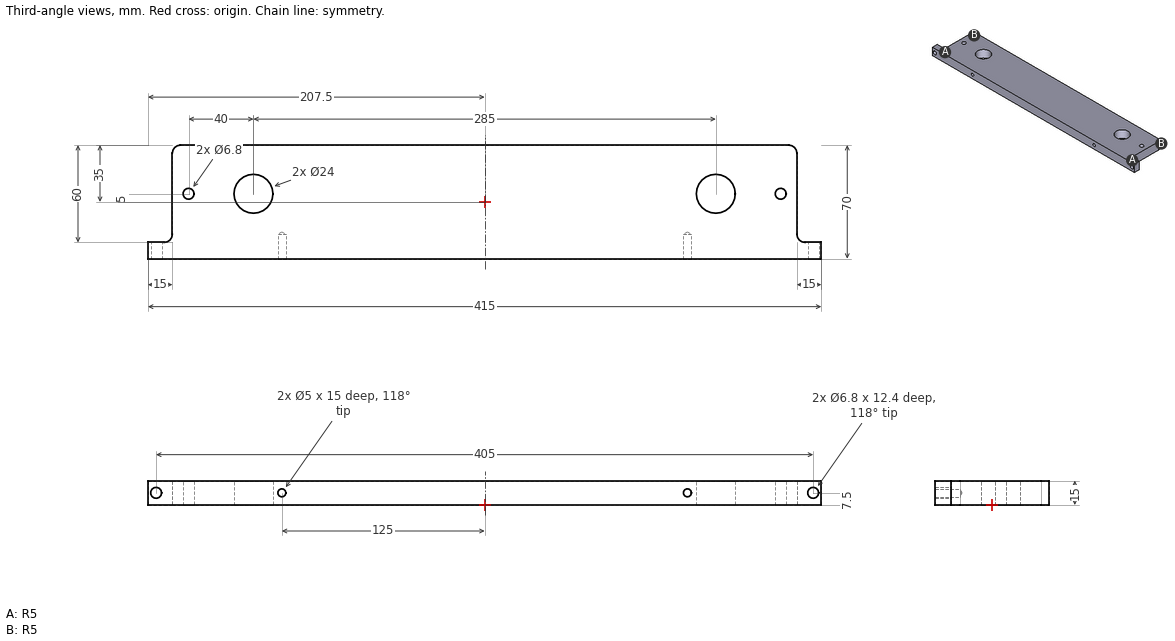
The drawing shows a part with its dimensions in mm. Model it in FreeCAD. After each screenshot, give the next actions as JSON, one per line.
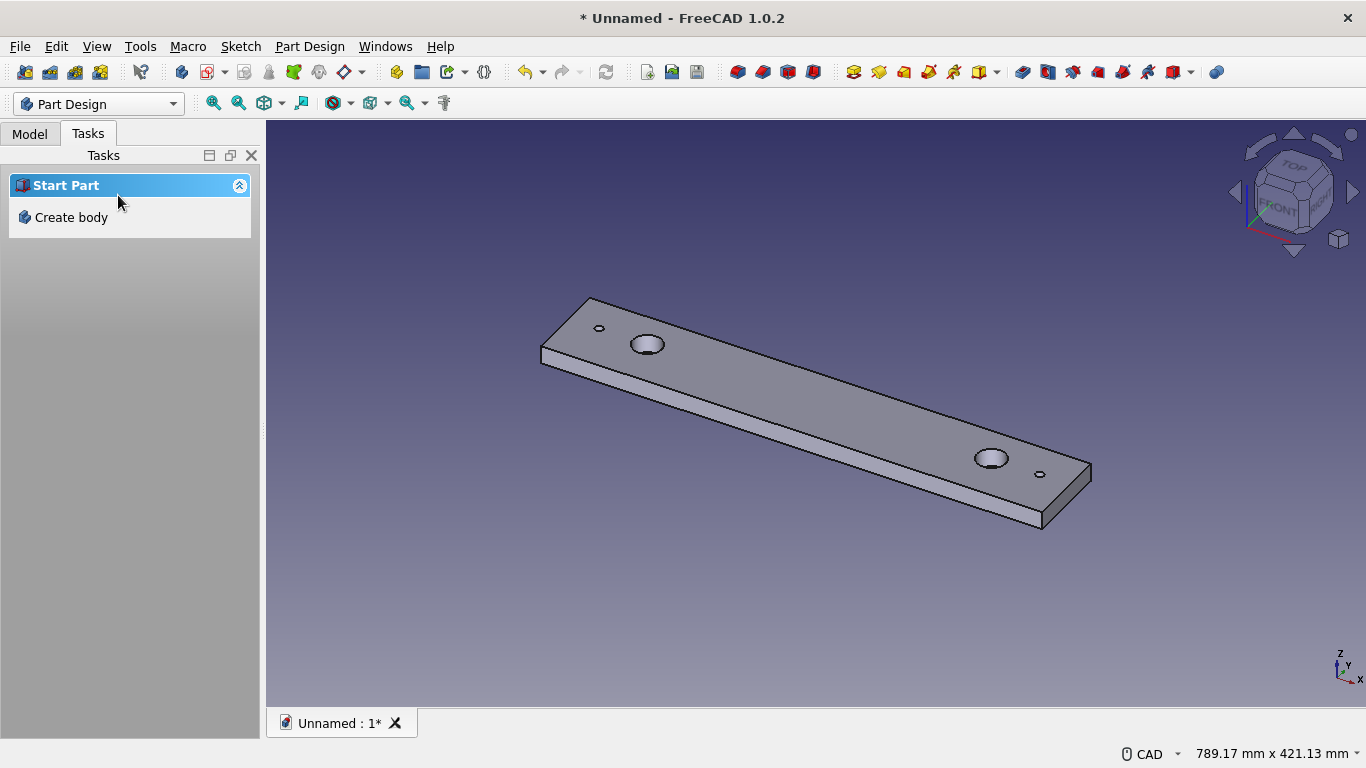
{"action": "left_click", "coordinate": [888, 428]}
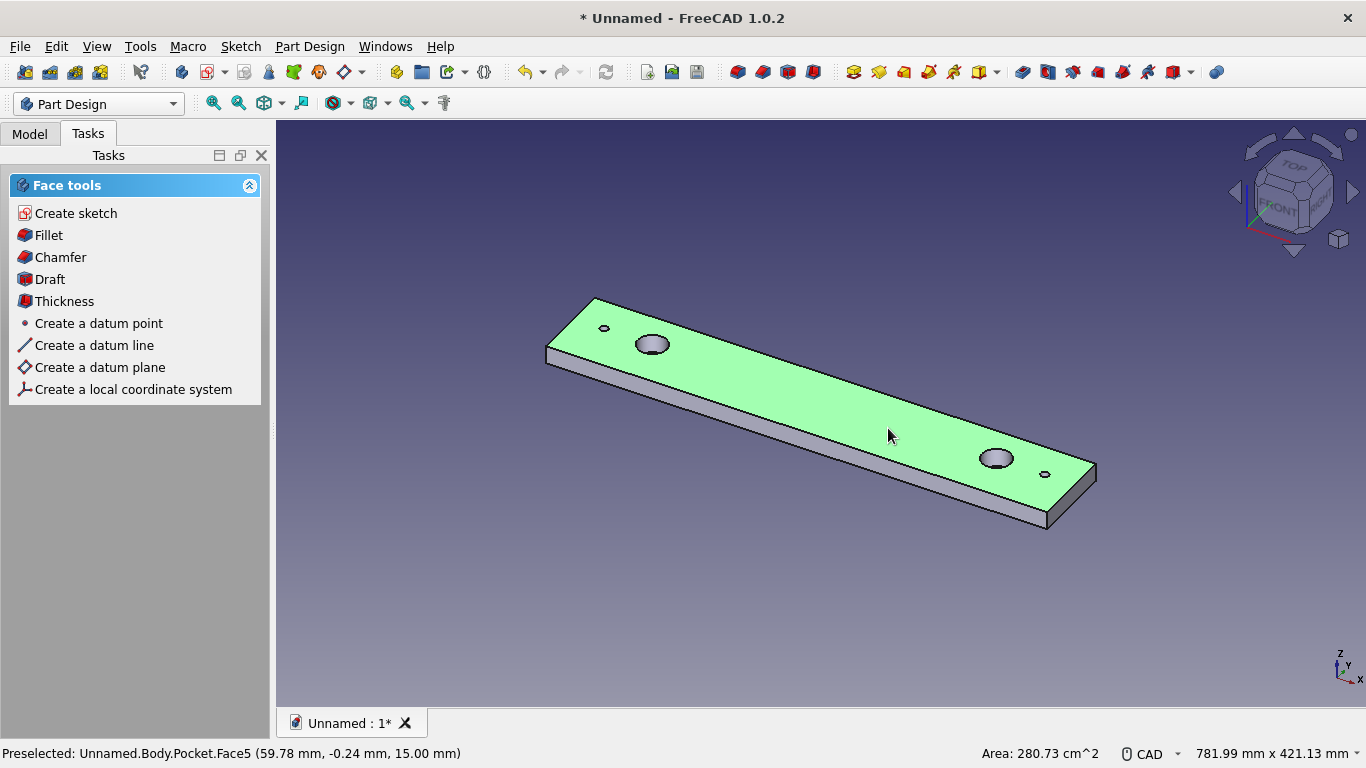
{"action": "left_click", "coordinate": [206, 72]}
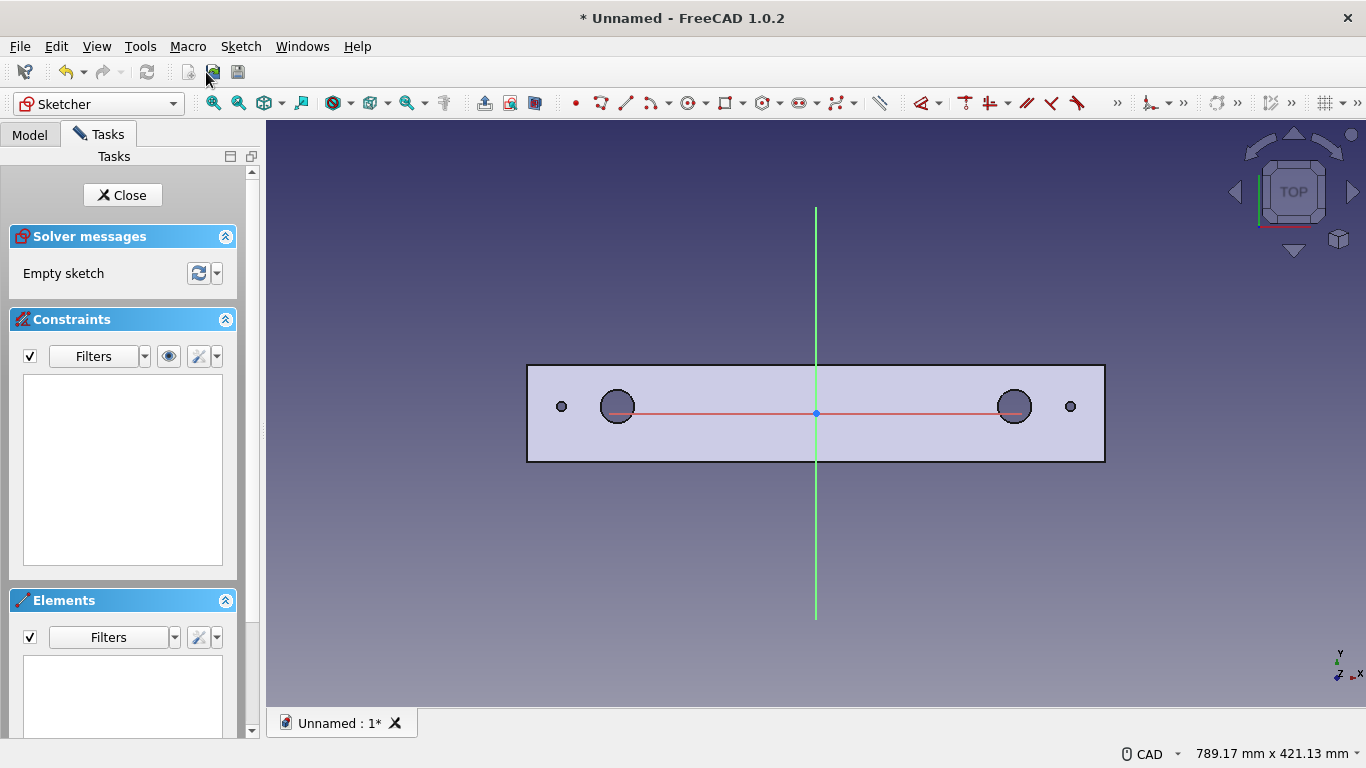
{"action": "left_click", "coordinate": [724, 104]}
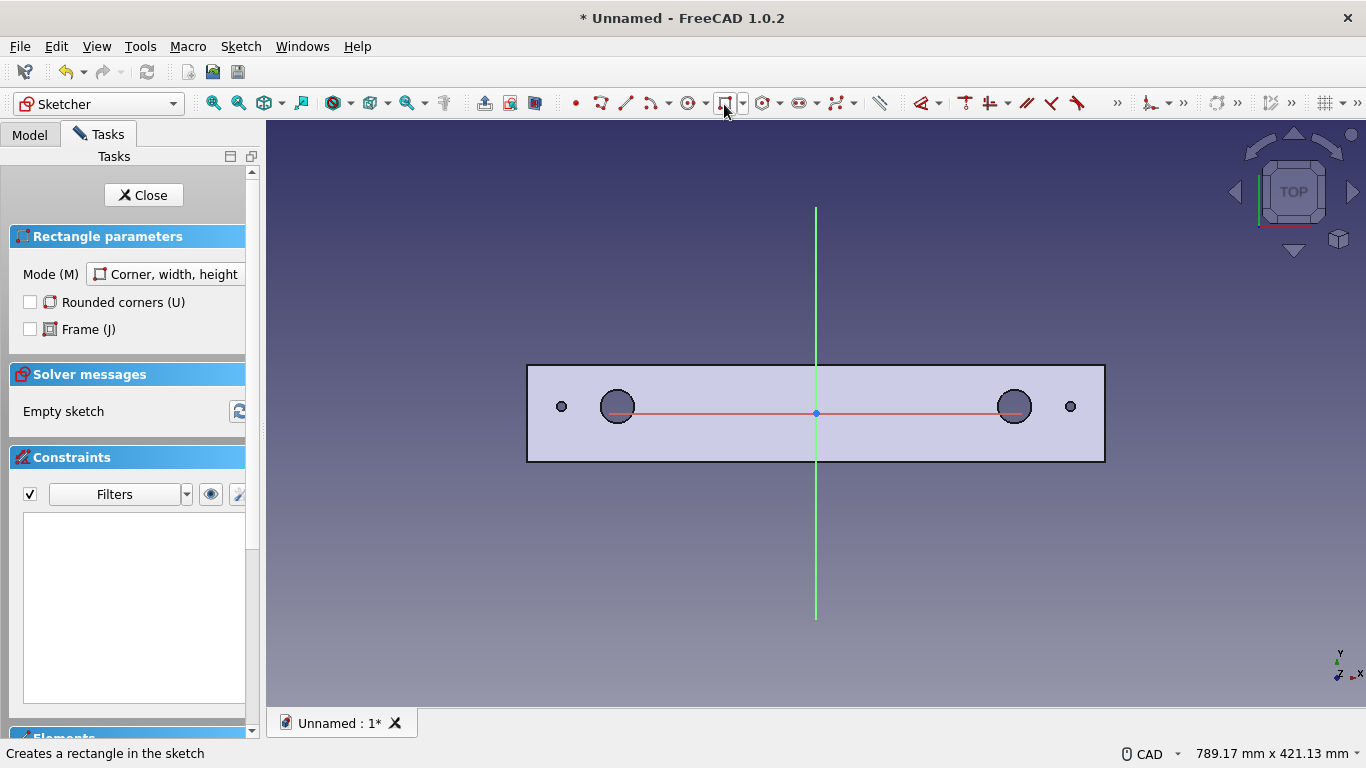
{"action": "left_click", "coordinate": [527, 365]}
{"action": "mouse_move", "coordinate": [548, 448]}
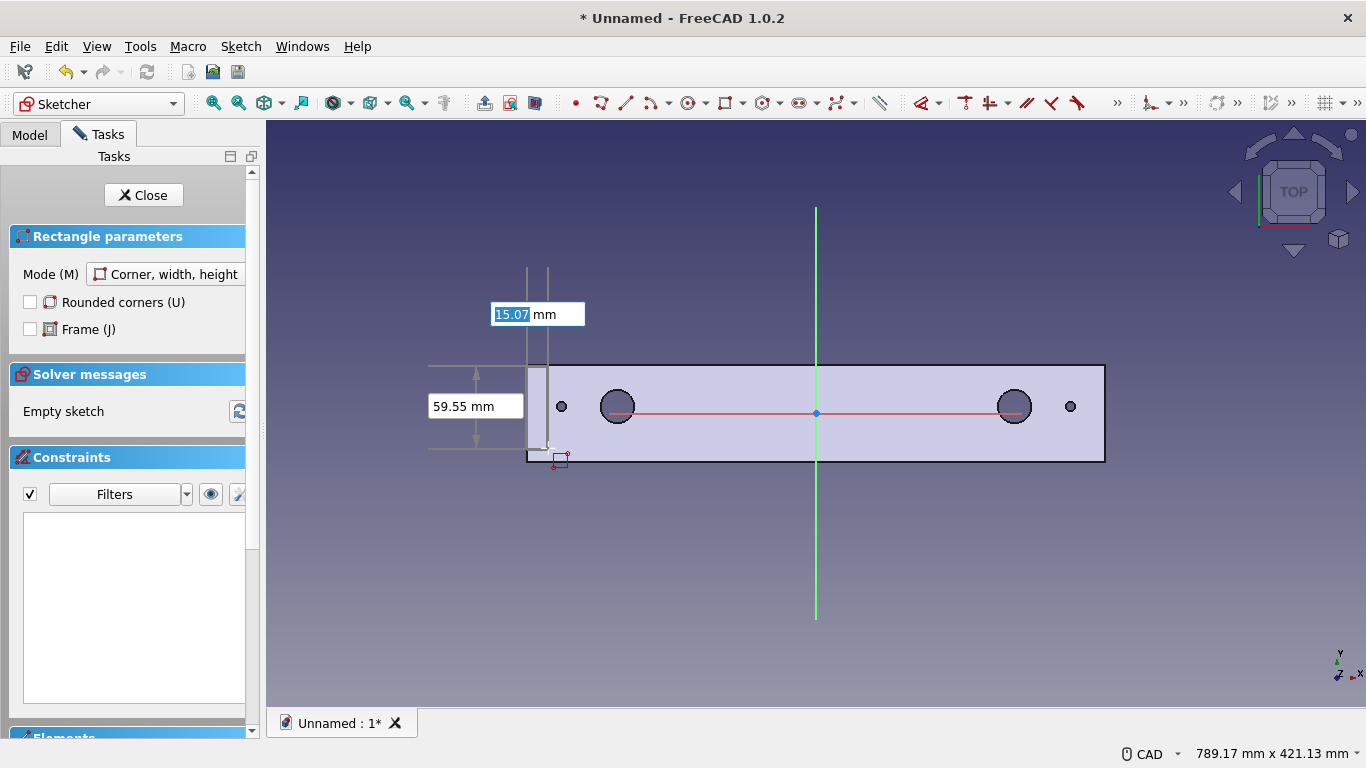
{"action": "type", "text": "15"}
{"action": "key", "text": "Tab"}
{"action": "type", "text": "60"}
{"action": "key", "text": "Return"}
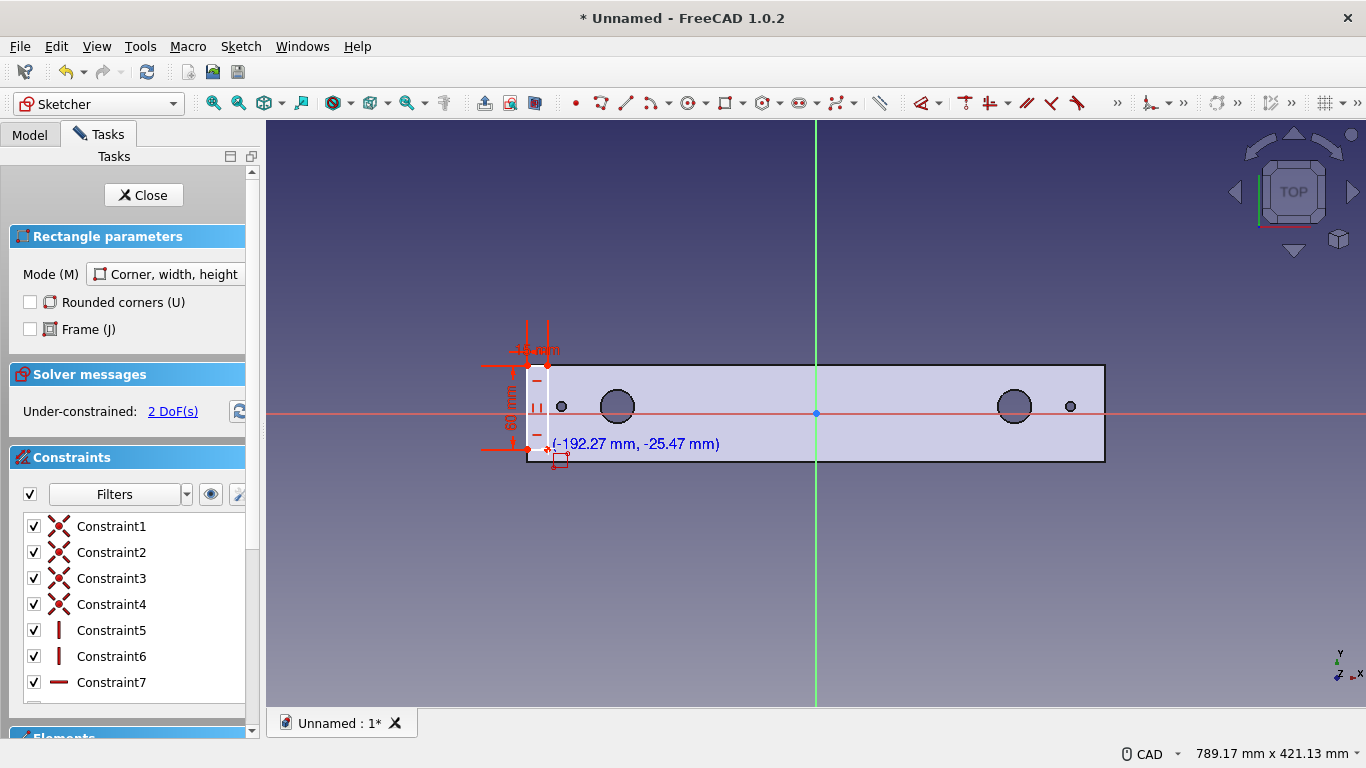
{"action": "left_click", "coordinate": [1084, 365]}
{"action": "mouse_move", "coordinate": [1105, 448]}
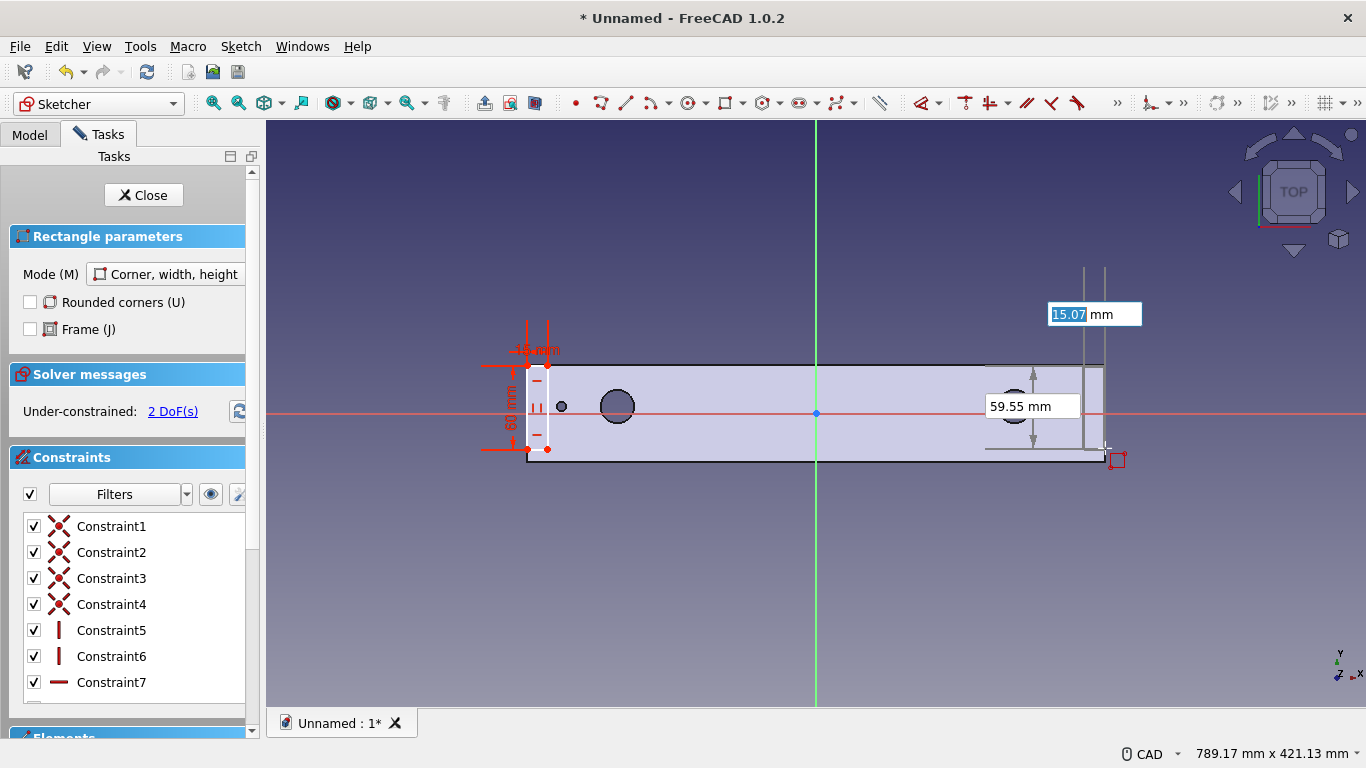
{"action": "type", "text": "15"}
{"action": "key", "text": "Tab"}
{"action": "type", "text": "60"}
{"action": "key", "text": "Return"}
{"action": "key", "text": "Escape"}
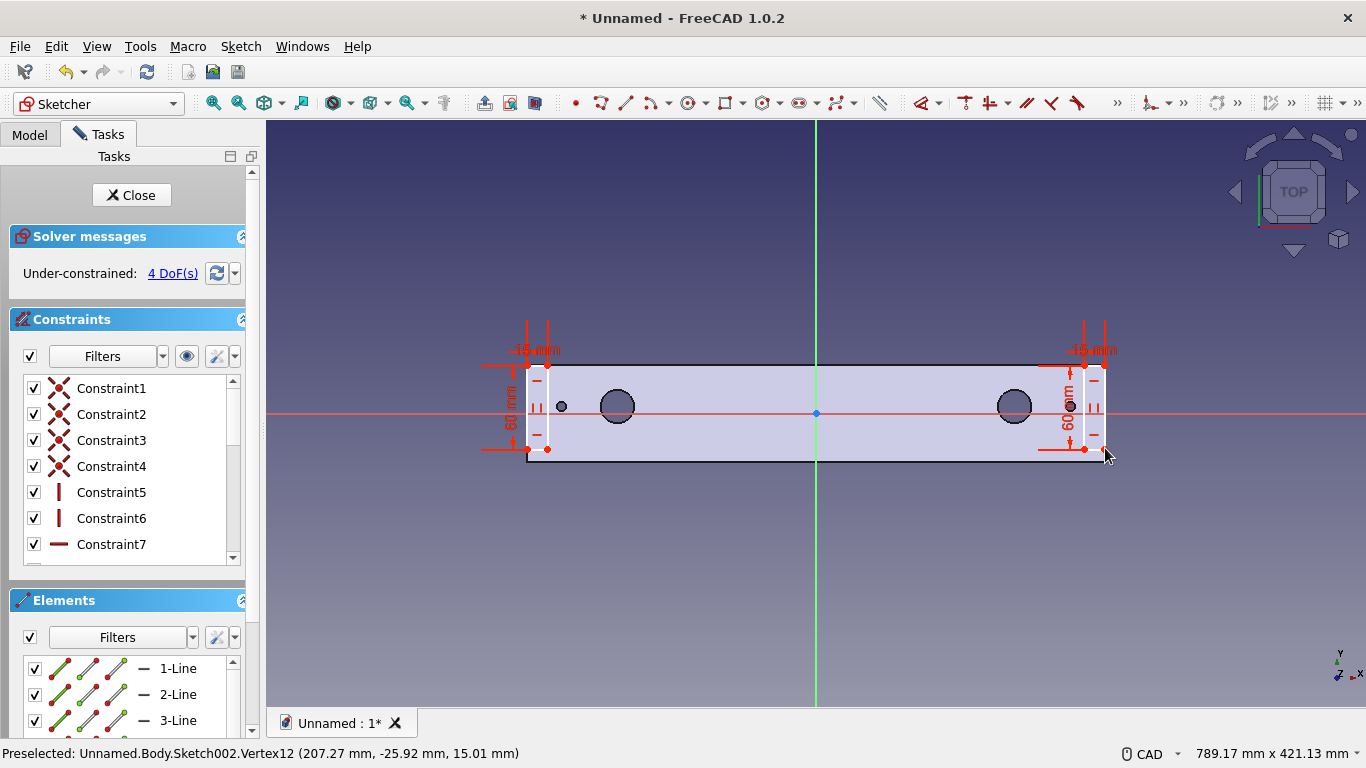
{"action": "left_click", "coordinate": [548, 366]}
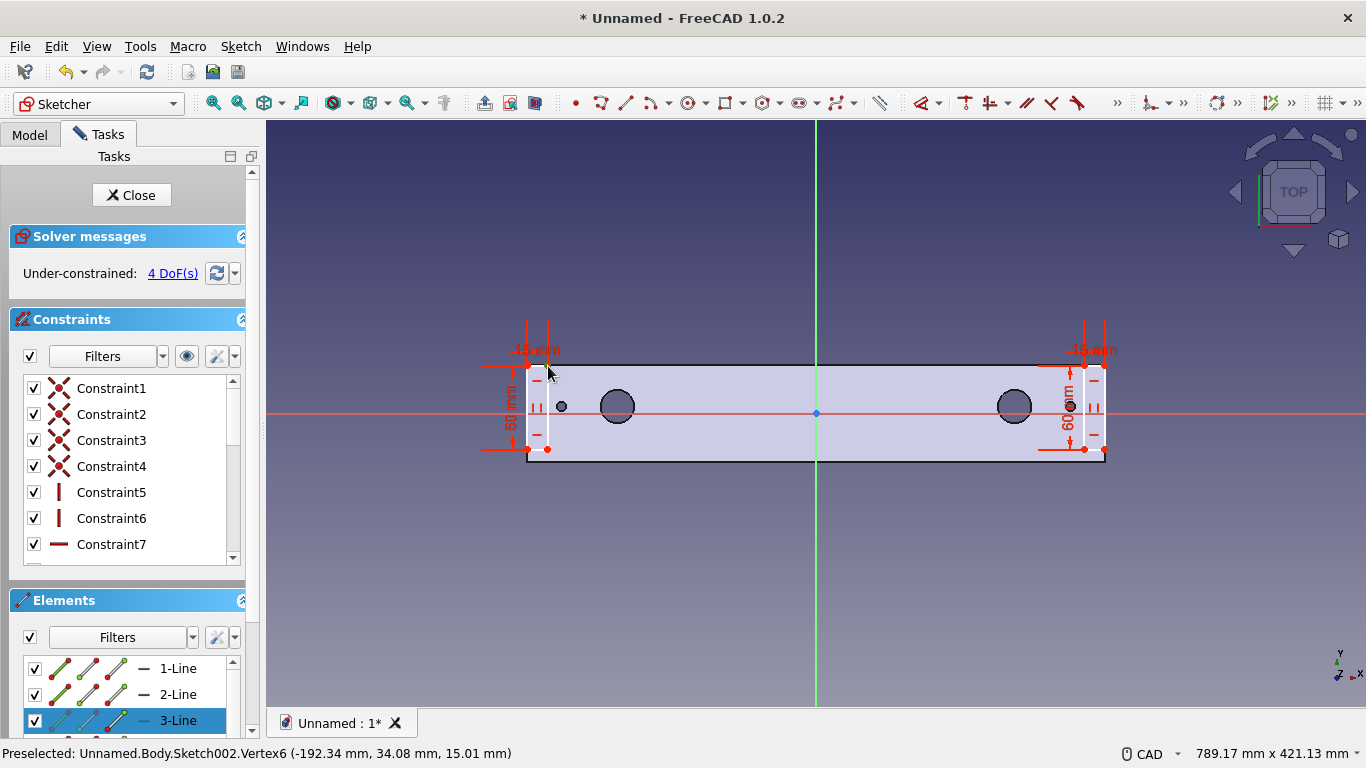
{"action": "left_click", "coordinate": [1084, 366]}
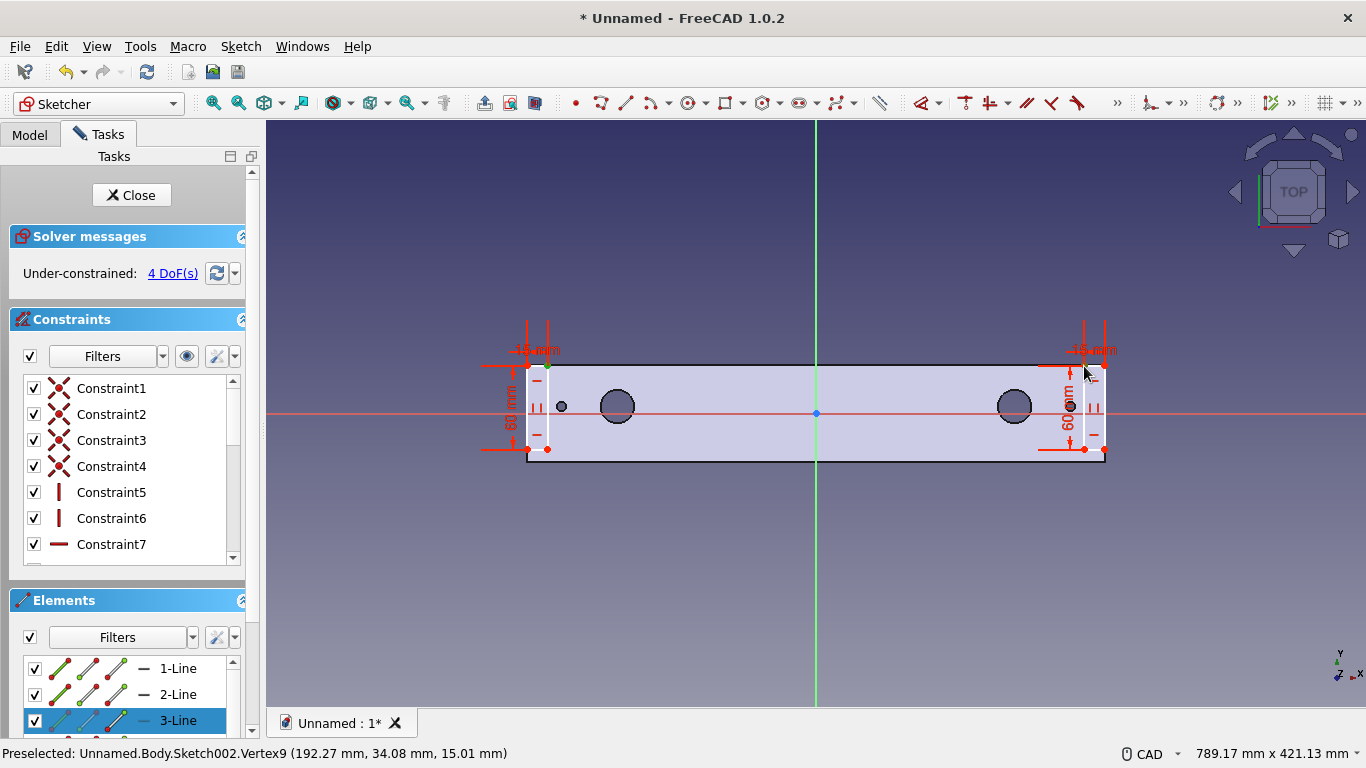
{"action": "left_click", "coordinate": [816, 641]}